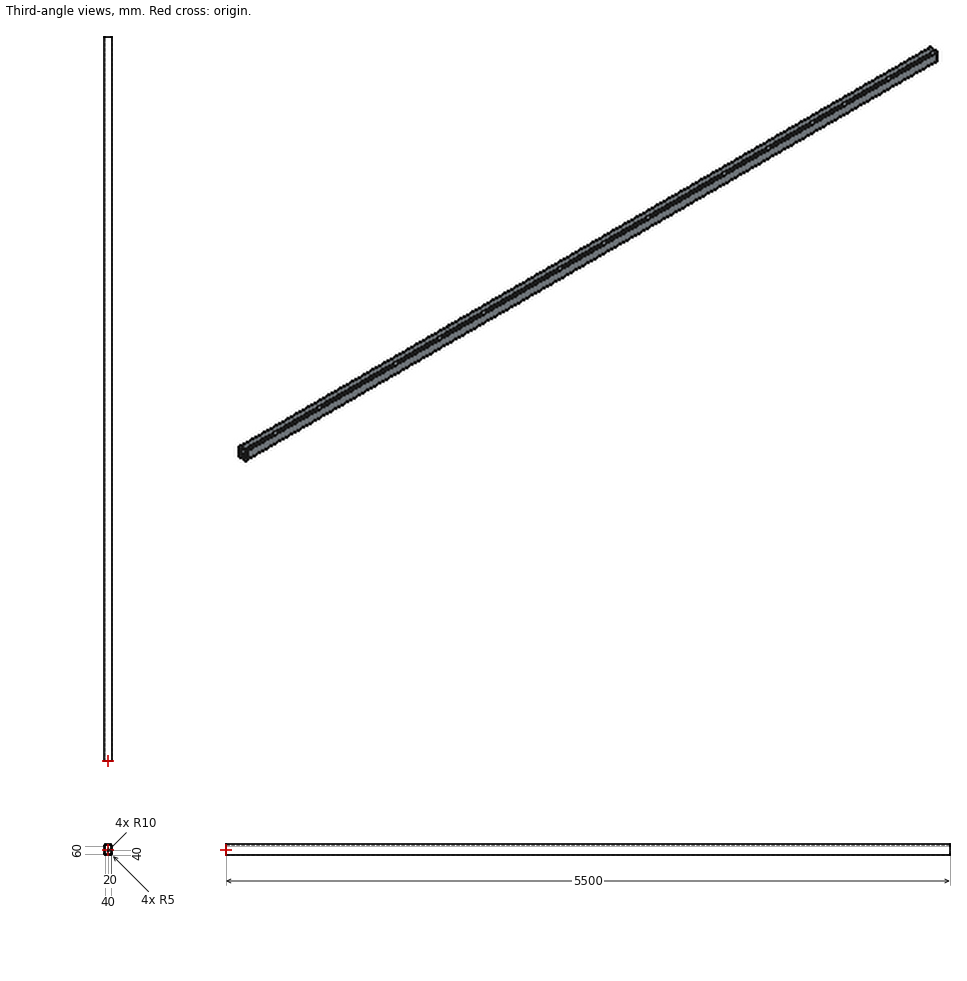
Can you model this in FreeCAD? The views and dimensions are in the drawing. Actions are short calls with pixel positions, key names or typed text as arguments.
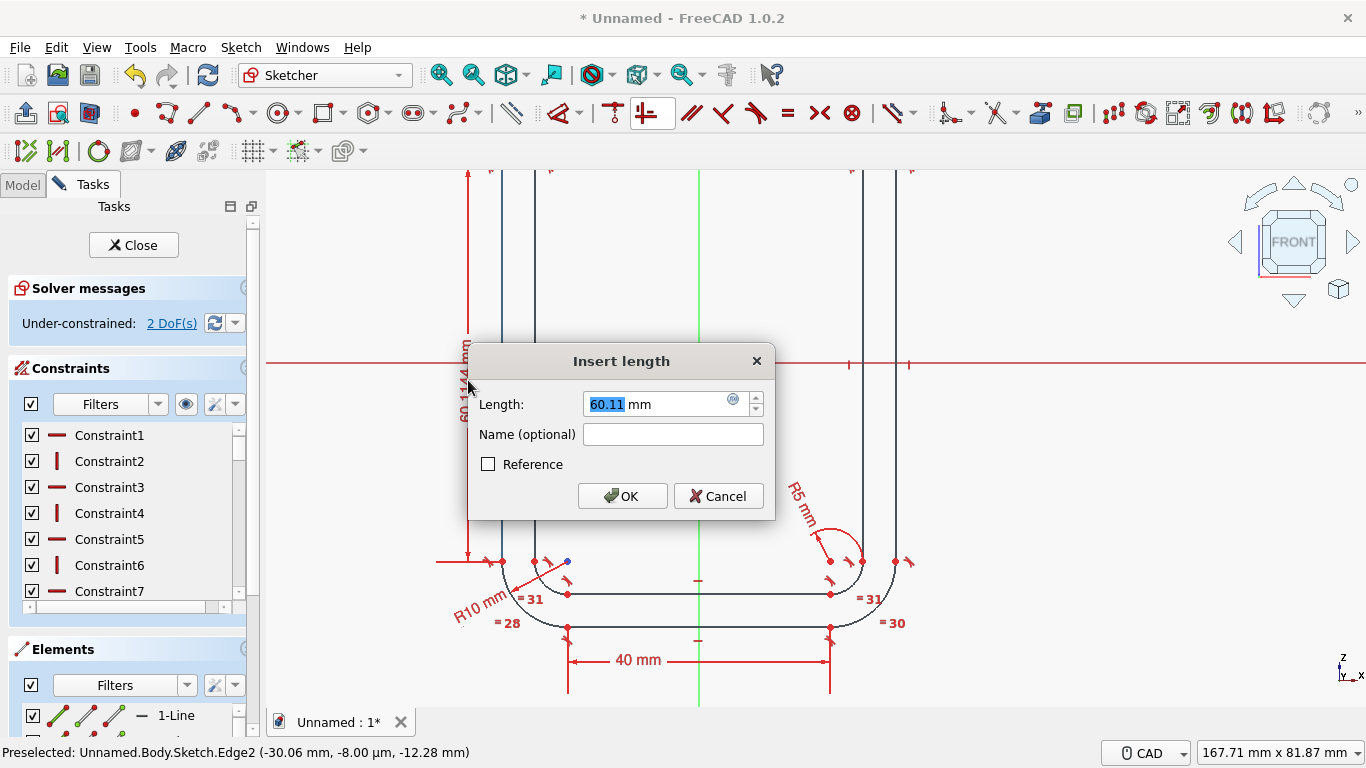
text(60)
key(Return)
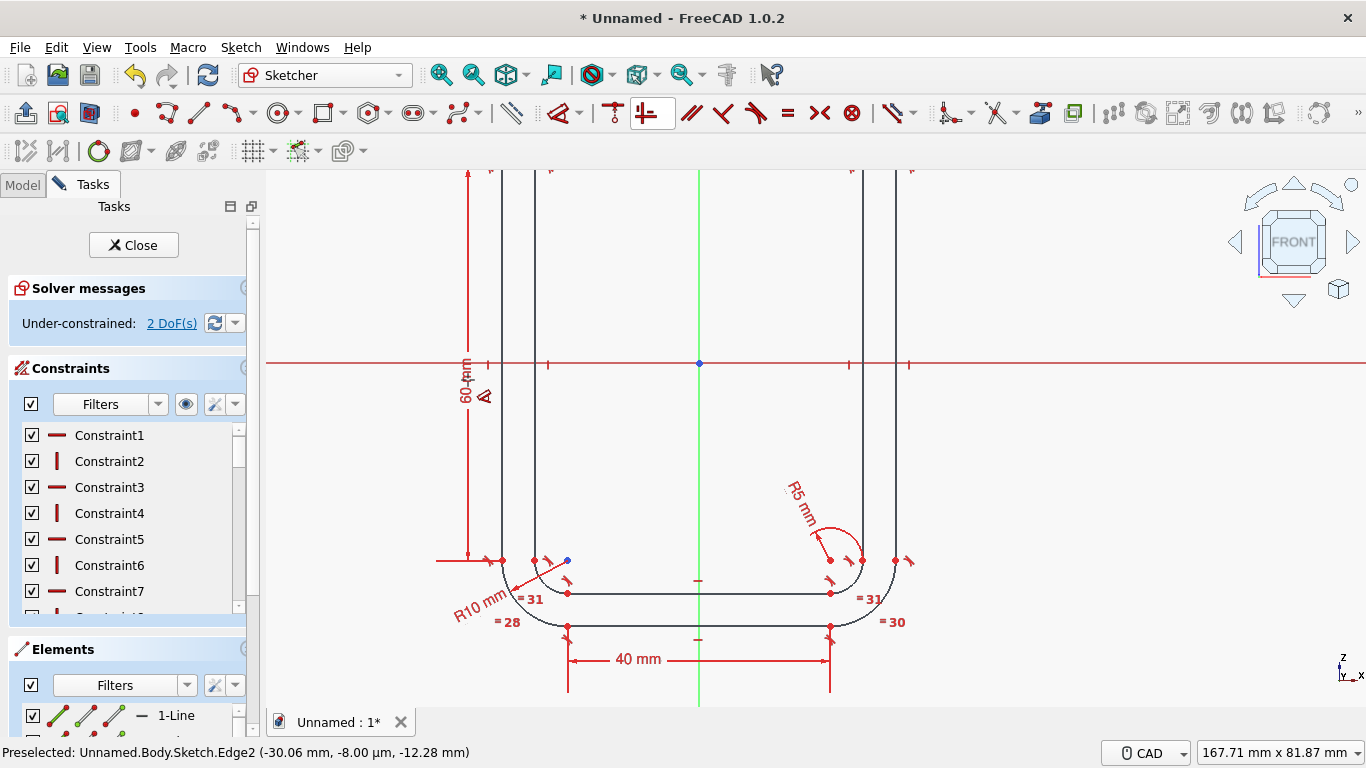
click(830, 626)
click(765, 660)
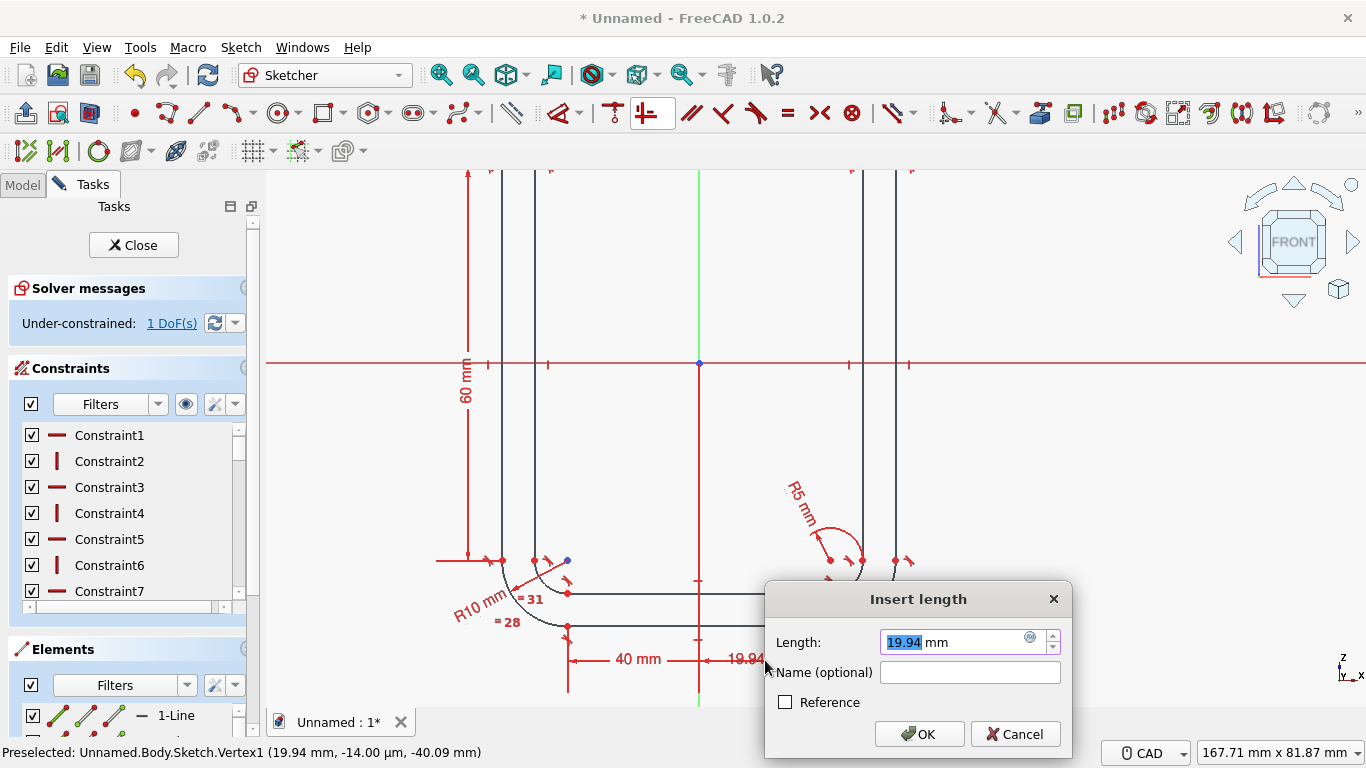
text(20)
key(Return)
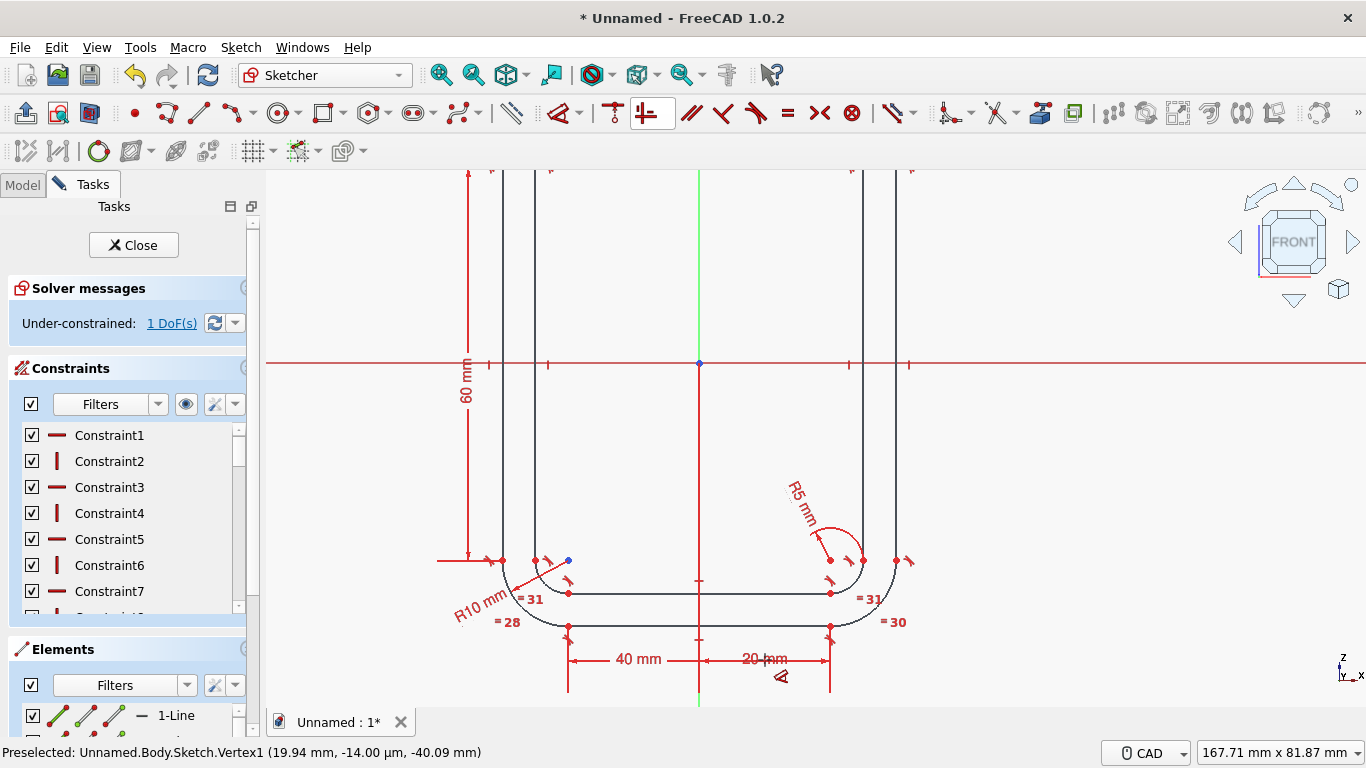
click(830, 626)
click(665, 495)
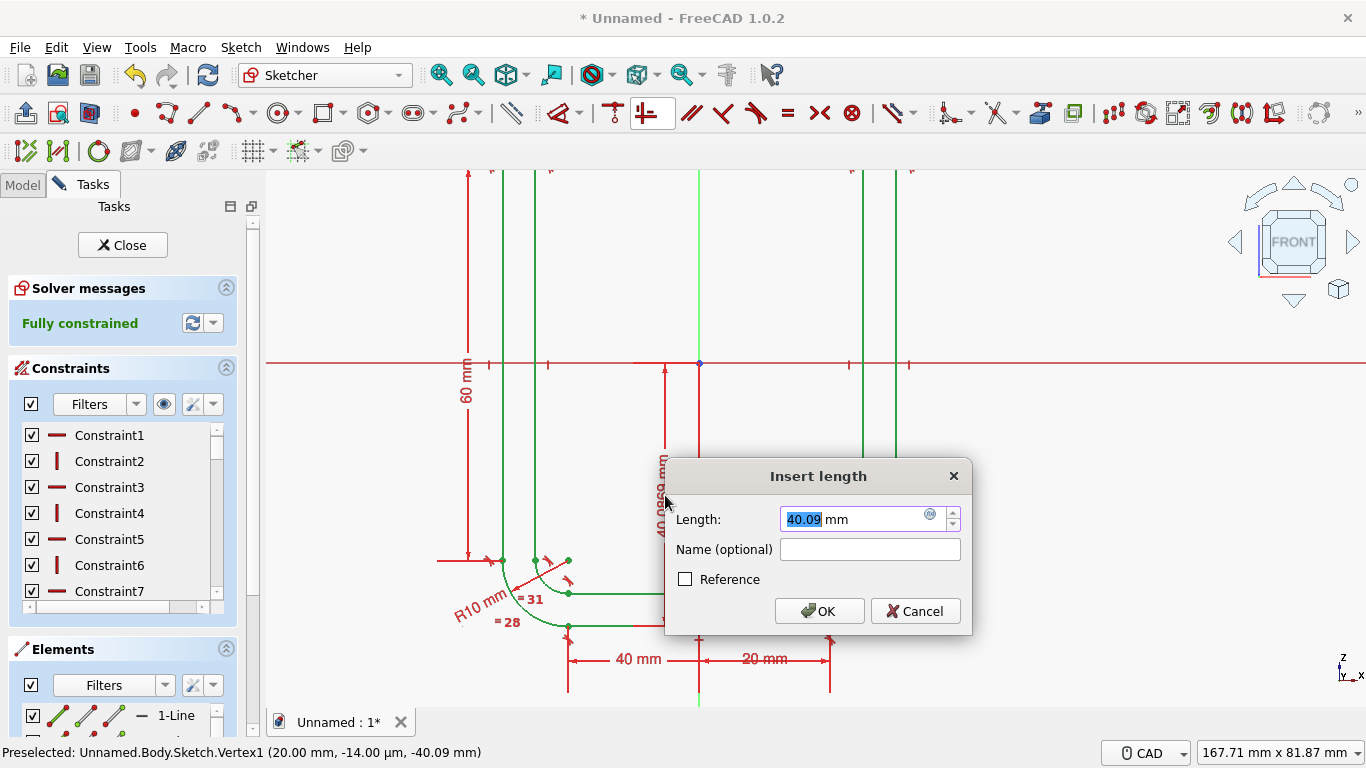
text(40)
key(Return)
key(Escape)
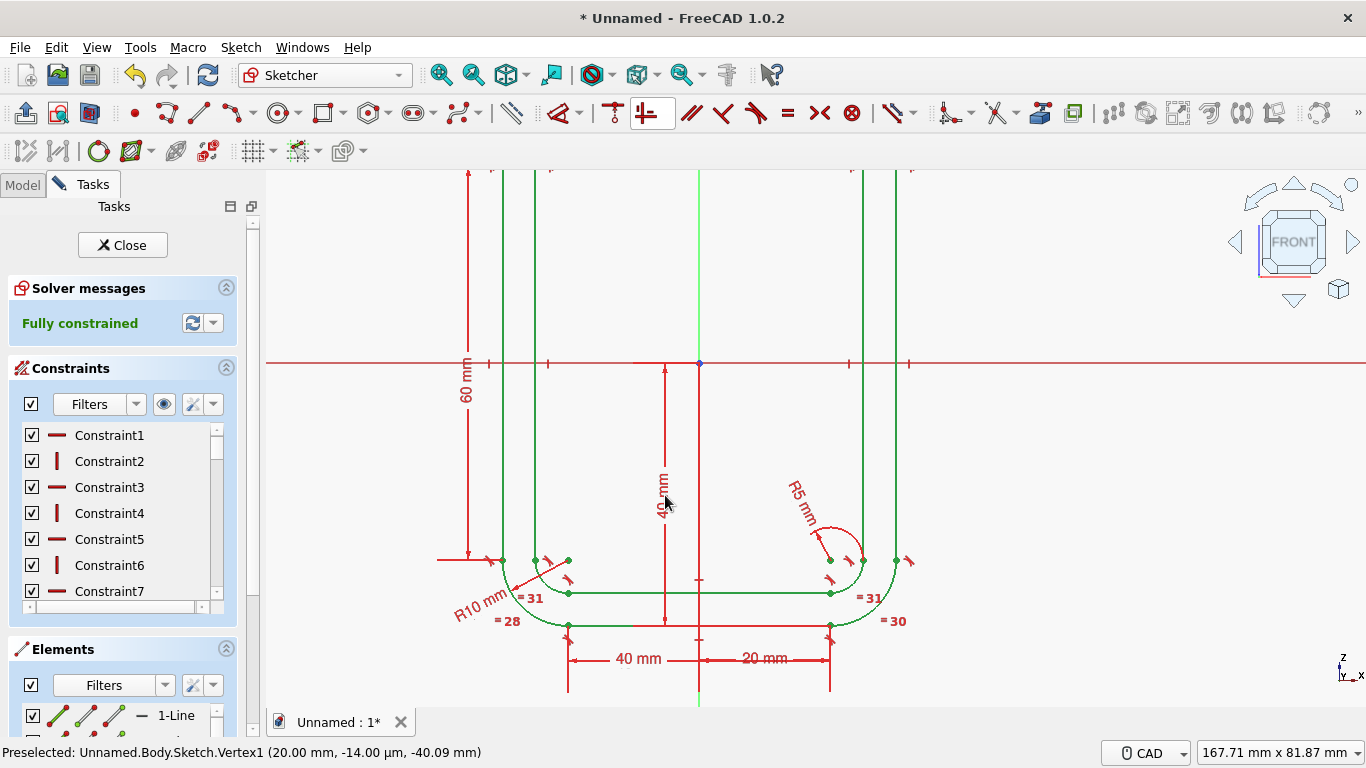
click(123, 245)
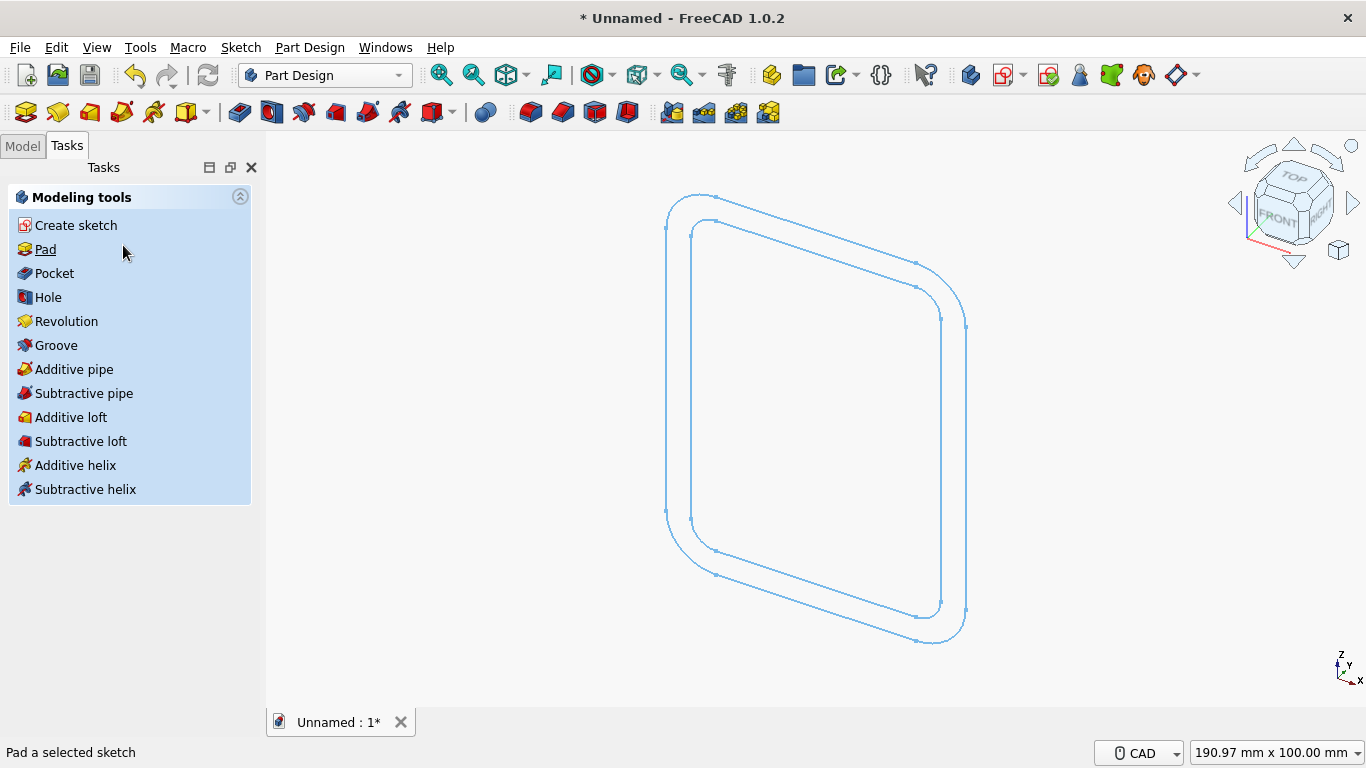
click(26, 112)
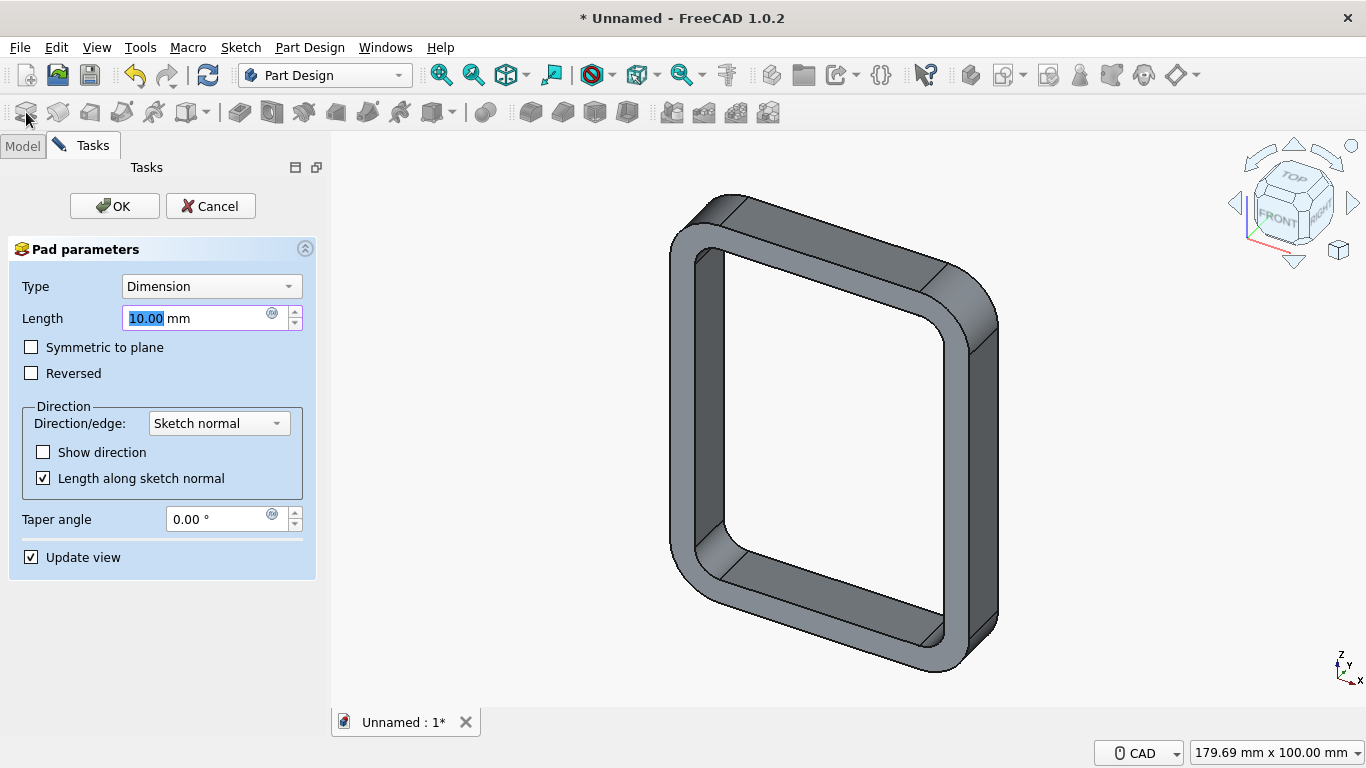
text(5500)
key(Tab)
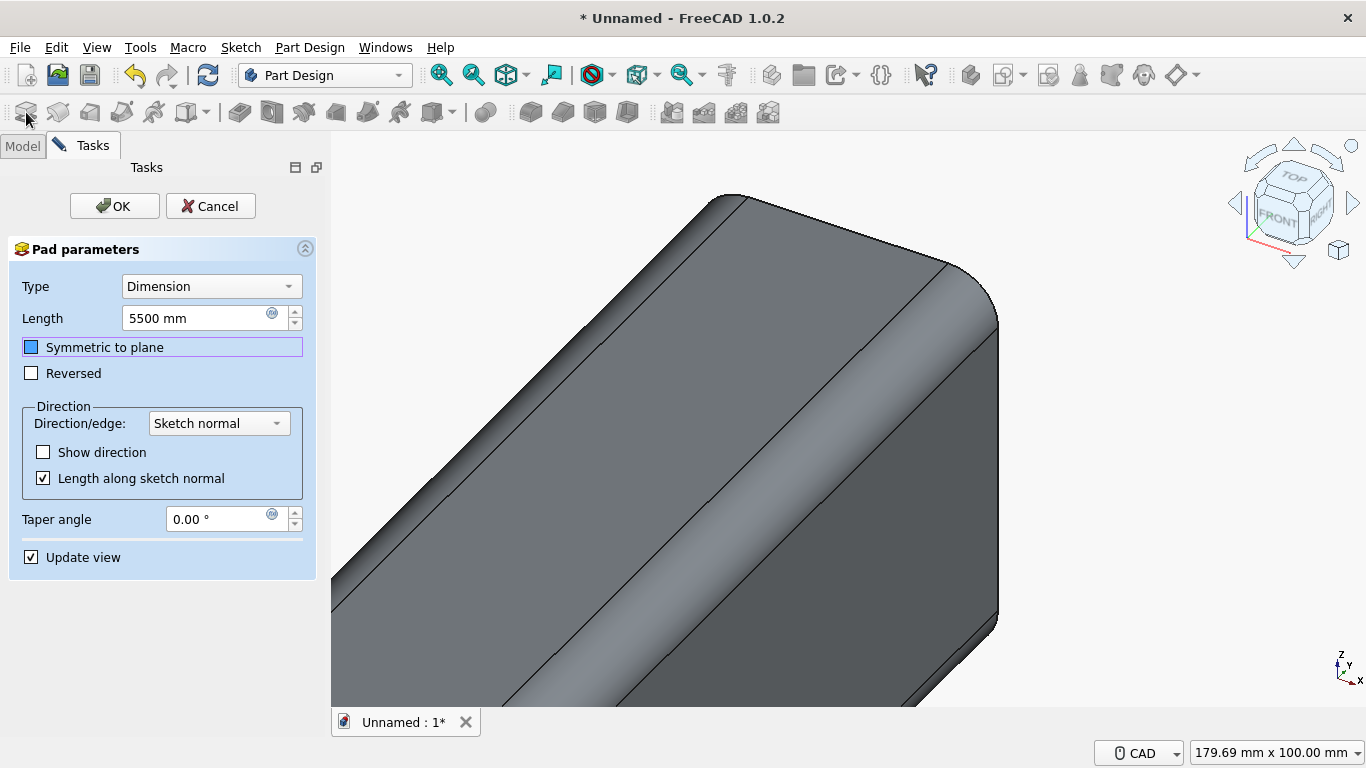
click(30, 373)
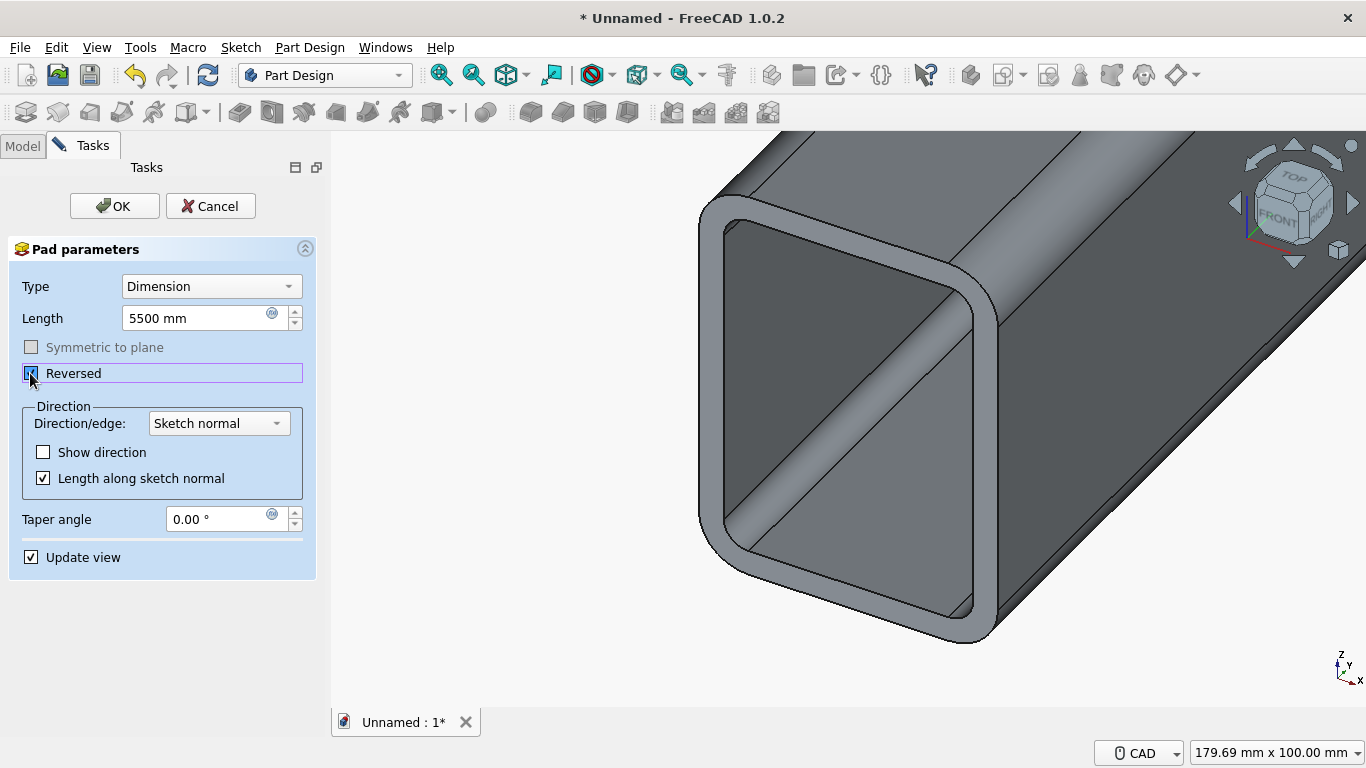
click(115, 206)